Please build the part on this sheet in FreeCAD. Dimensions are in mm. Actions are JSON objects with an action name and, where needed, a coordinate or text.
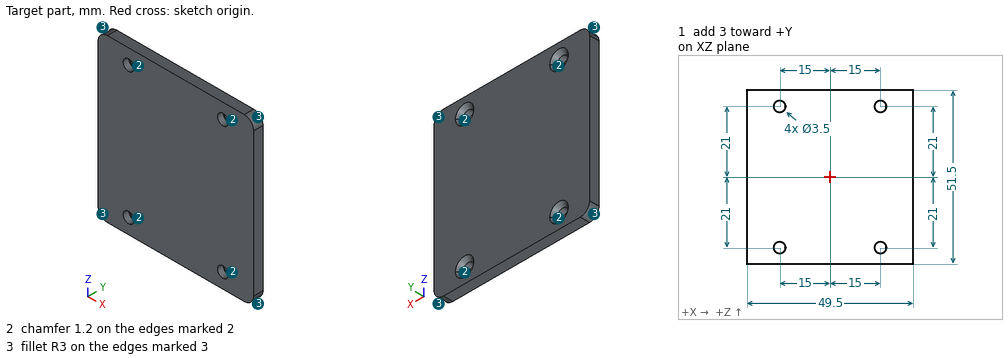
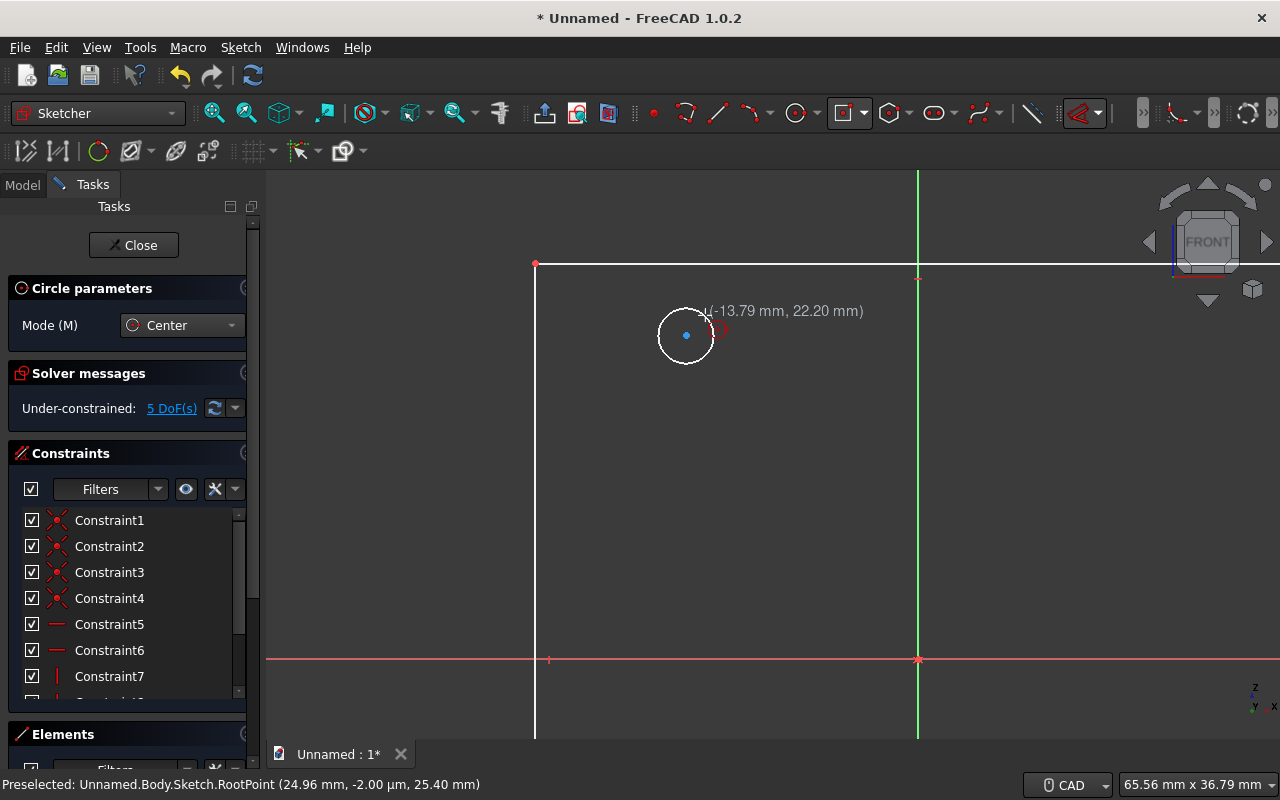
{"action": "scroll", "coordinate": [530, 287], "scroll_direction": "down", "scroll_amount": 4}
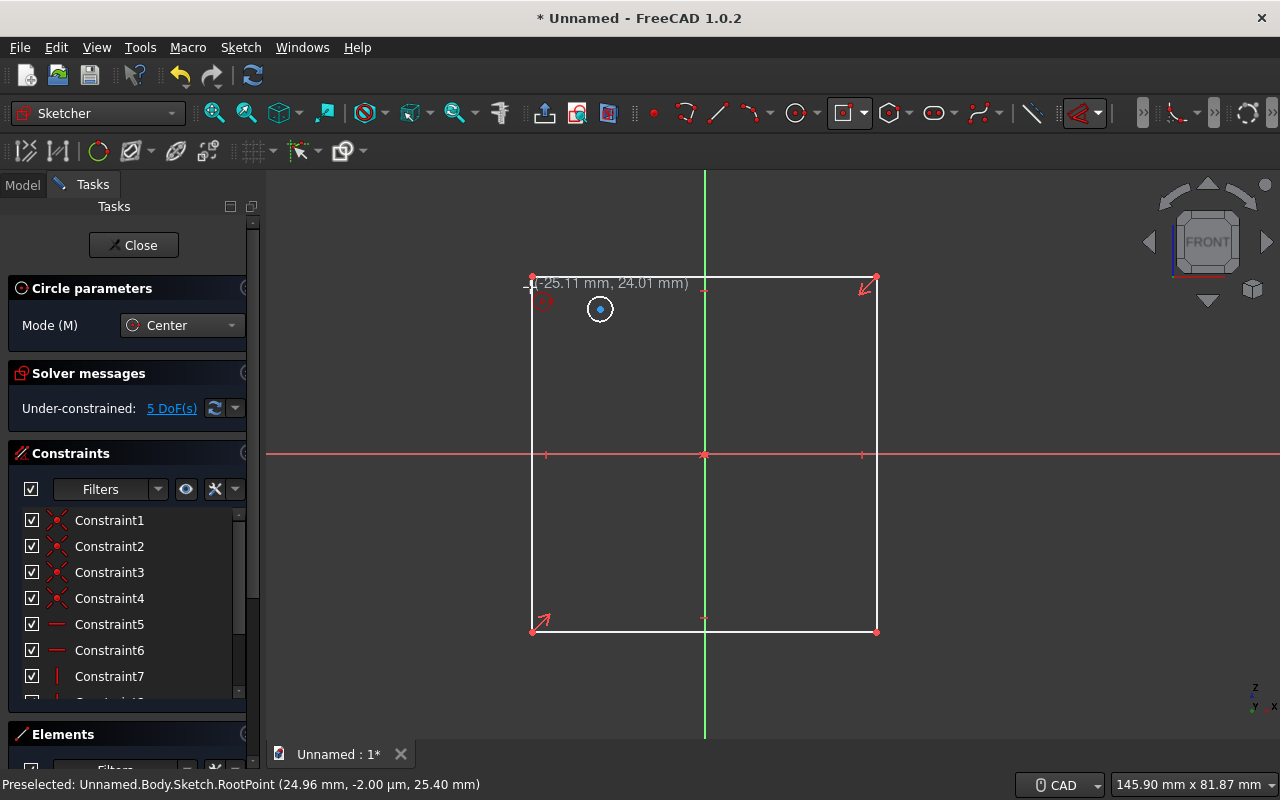
{"action": "scroll", "coordinate": [809, 308], "scroll_direction": "up", "scroll_amount": 4}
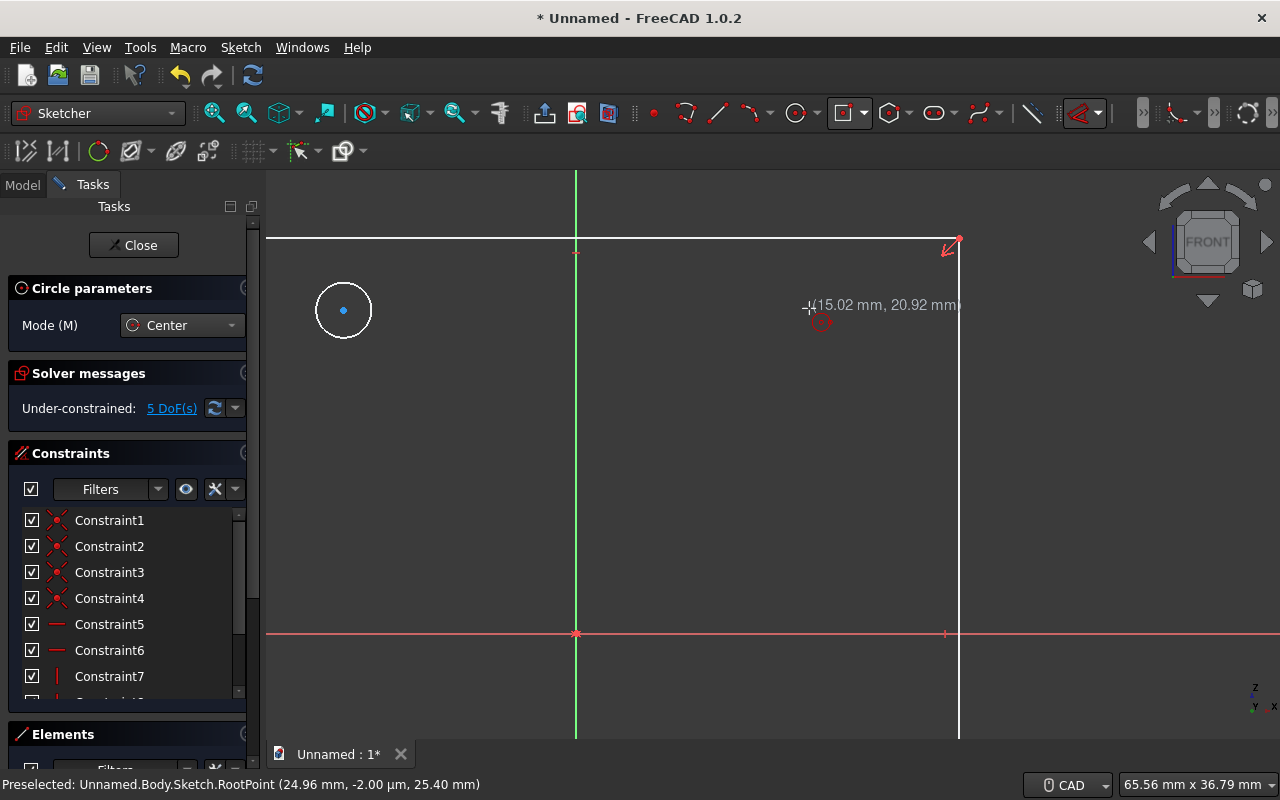
{"action": "left_click", "coordinate": [808, 309]}
{"action": "left_click", "coordinate": [827, 290]}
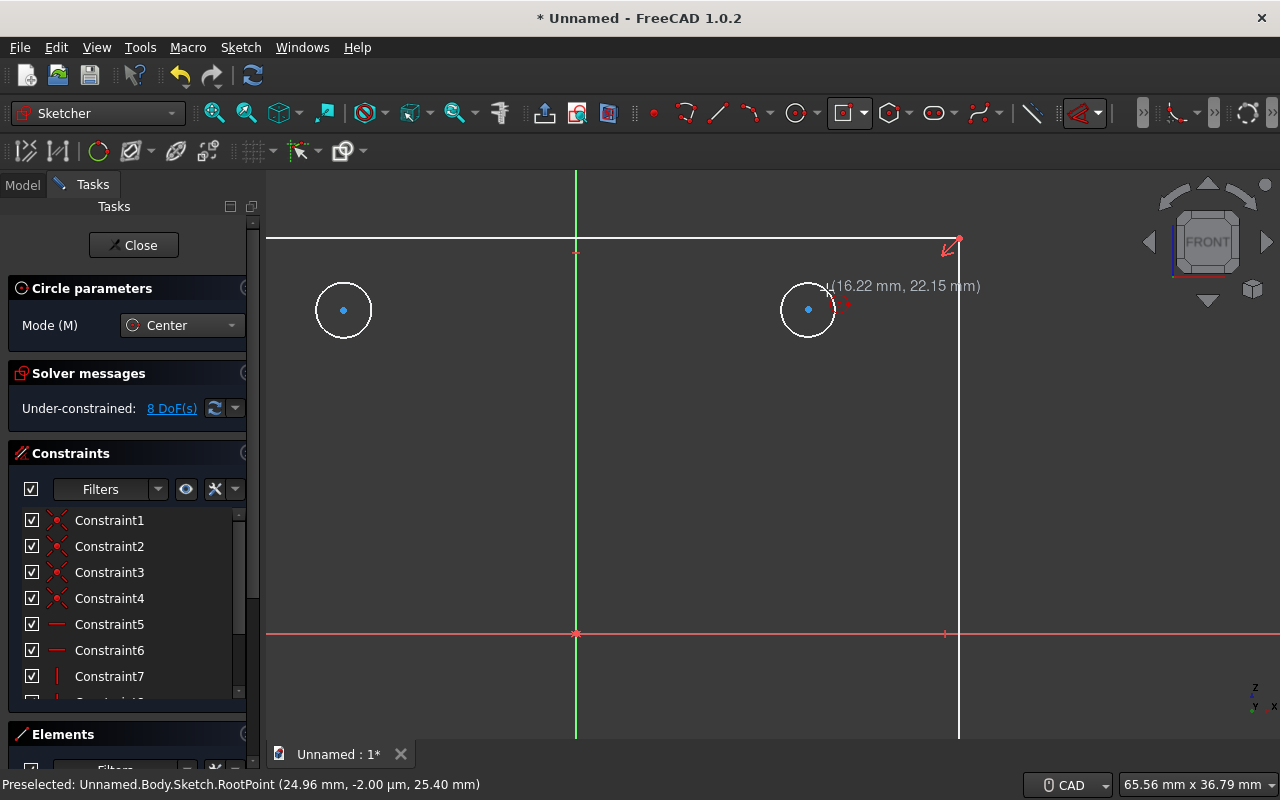
{"action": "scroll", "coordinate": [809, 308], "scroll_direction": "down", "scroll_amount": 4}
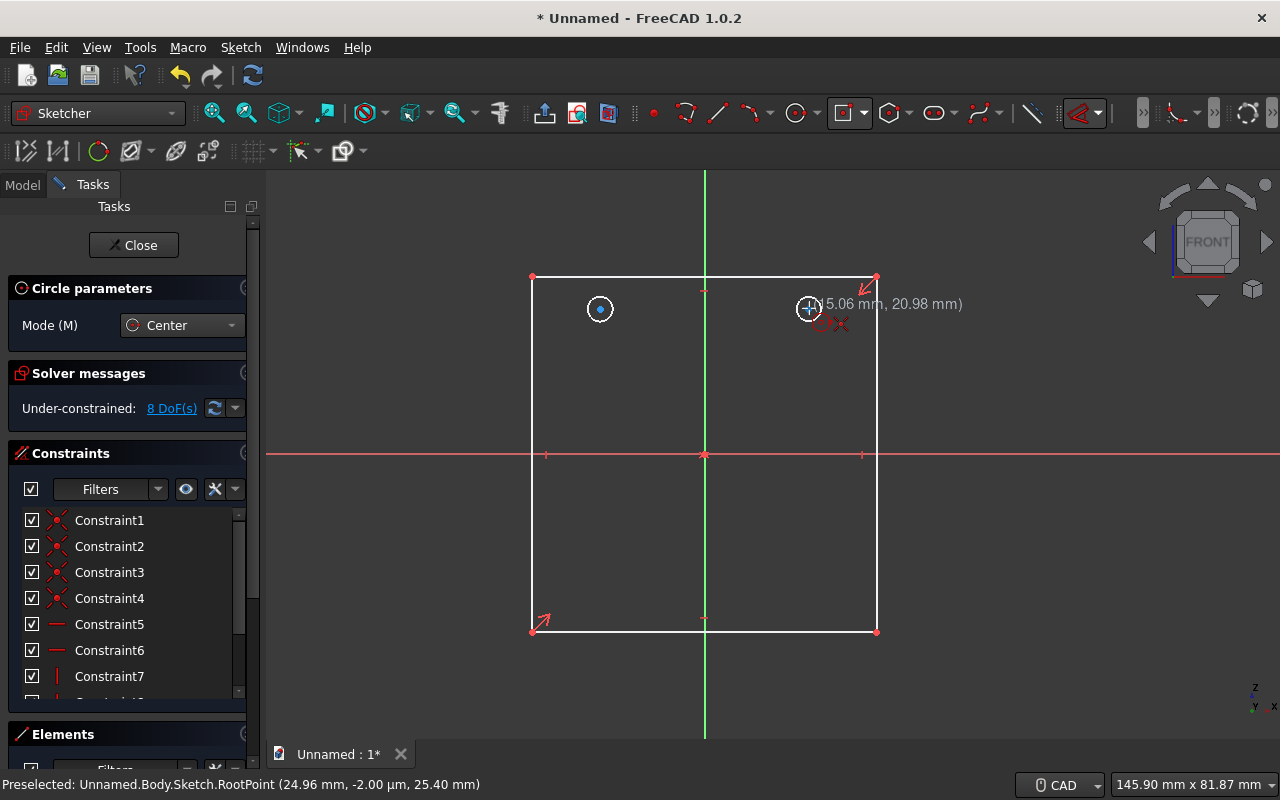
{"action": "scroll", "coordinate": [600, 600], "scroll_direction": "up", "scroll_amount": 4}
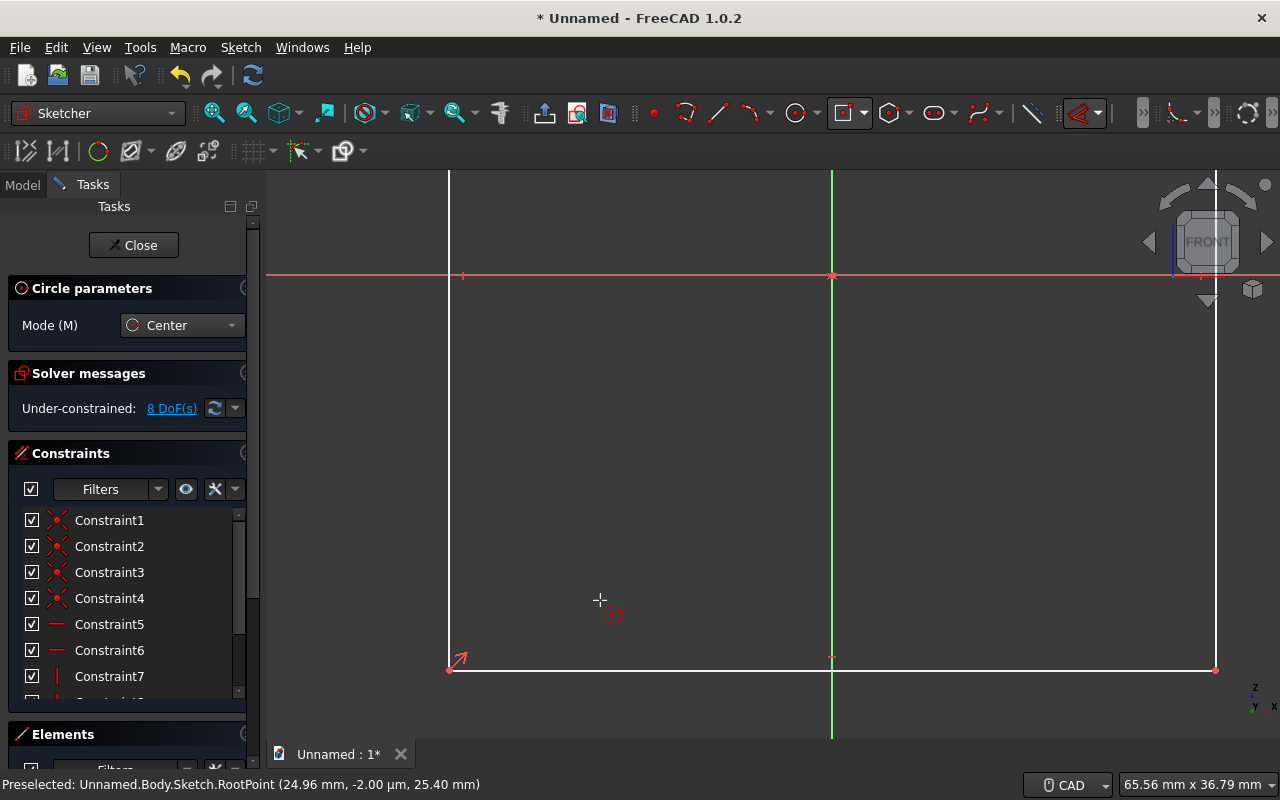
{"action": "left_click", "coordinate": [600, 600]}
{"action": "left_click", "coordinate": [620, 581]}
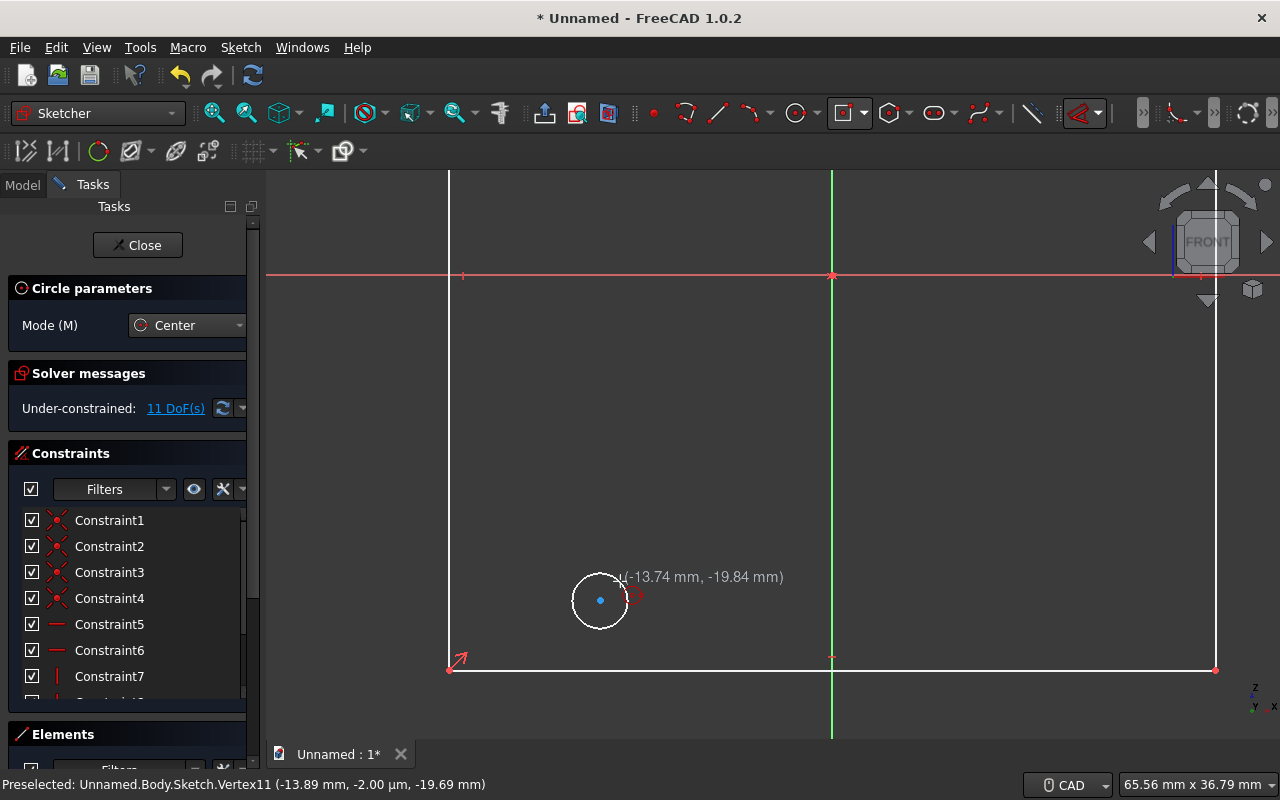
{"action": "left_click", "coordinate": [1064, 600]}
{"action": "left_click", "coordinate": [1084, 581]}
{"action": "key", "text": "Escape"}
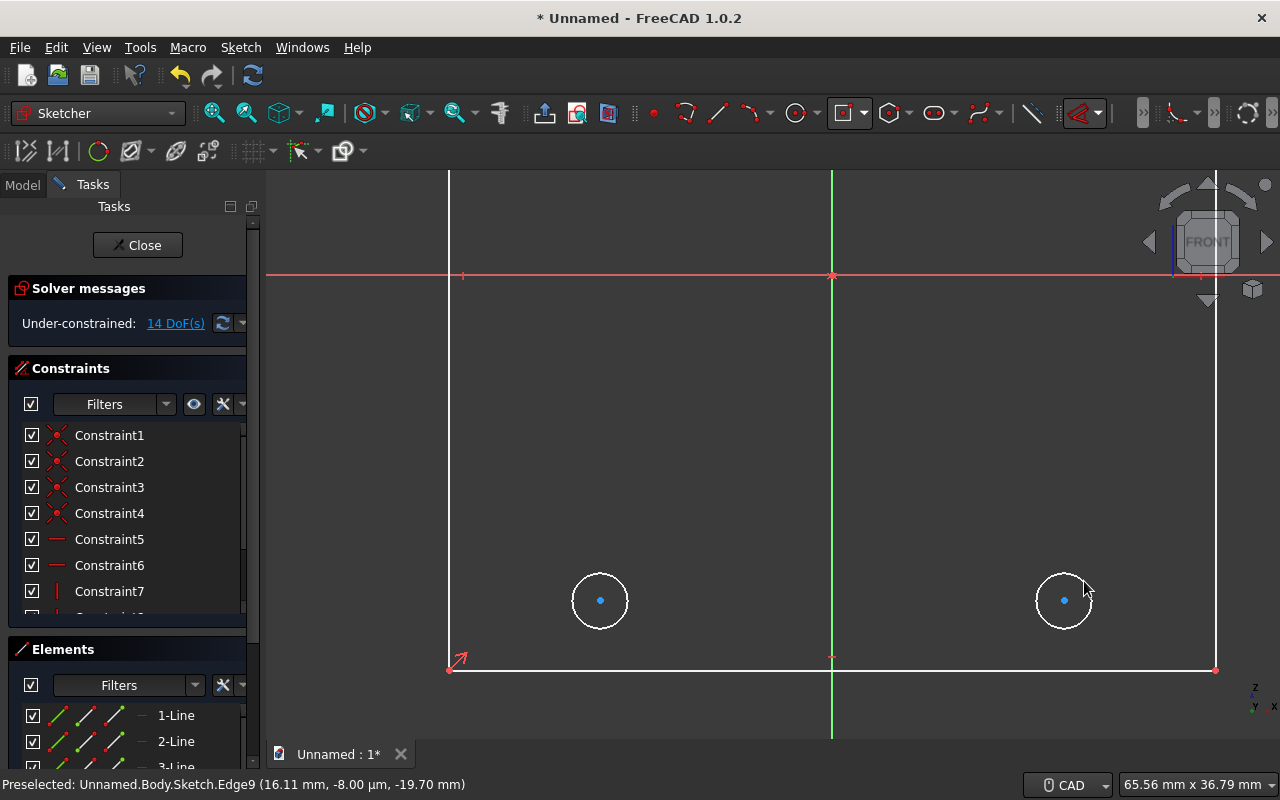
{"action": "scroll", "coordinate": [600, 601], "scroll_direction": "down", "scroll_amount": 4}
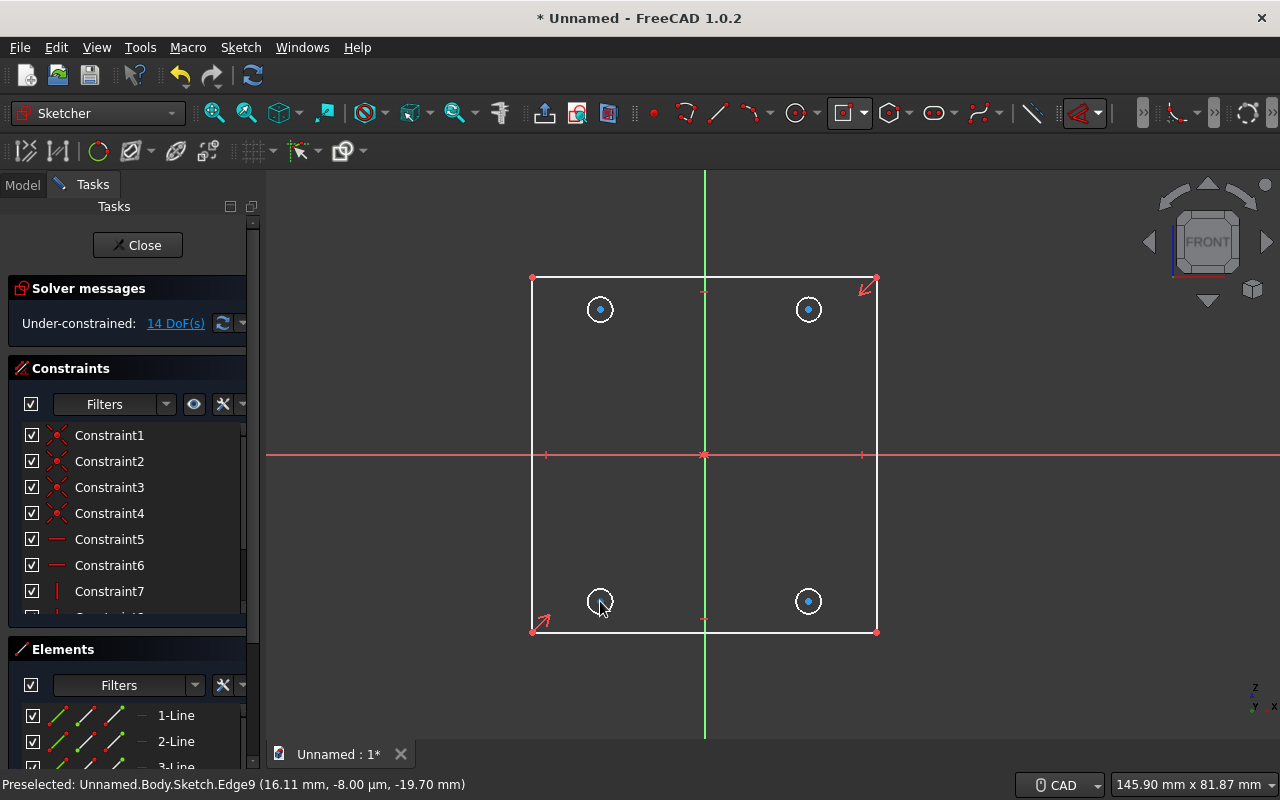
{"action": "left_click", "coordinate": [609, 301]}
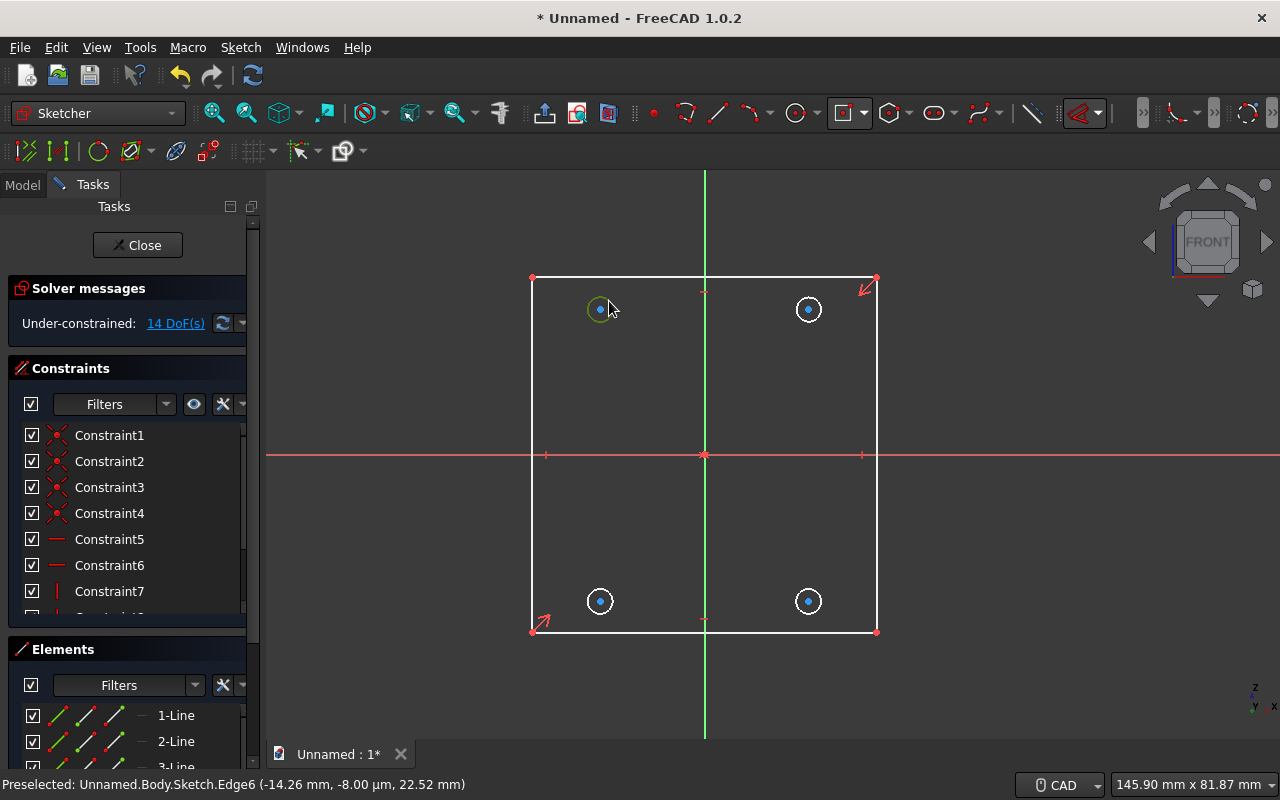
{"action": "left_click", "coordinate": [817, 301]}